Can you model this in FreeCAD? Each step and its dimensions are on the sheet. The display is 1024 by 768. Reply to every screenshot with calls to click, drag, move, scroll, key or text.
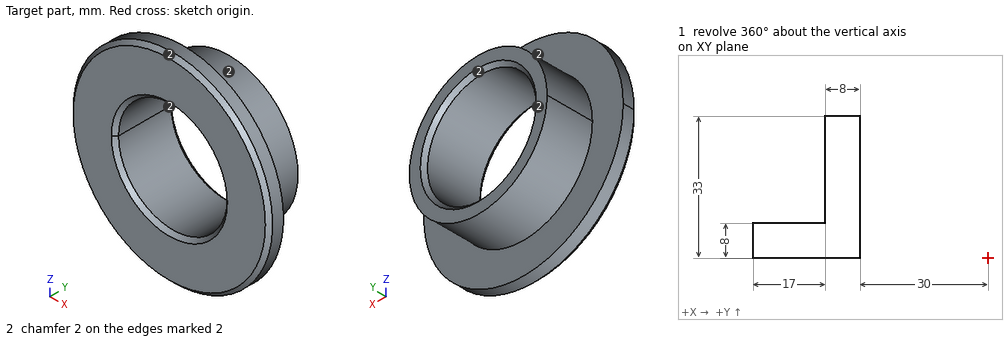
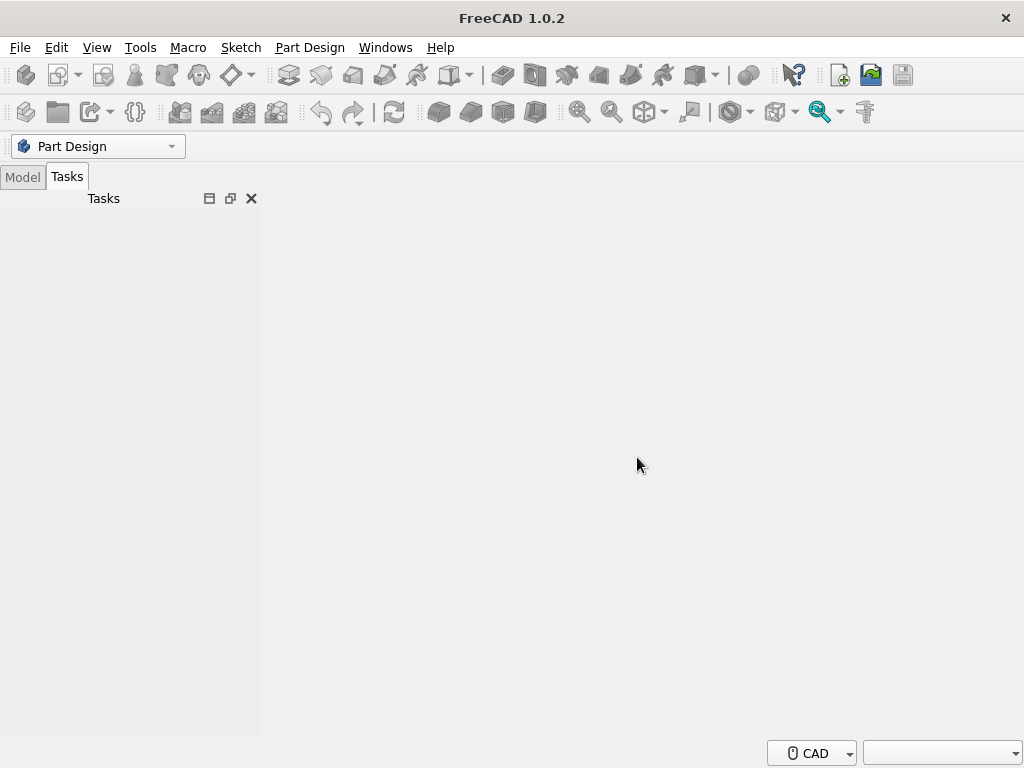
click(840, 76)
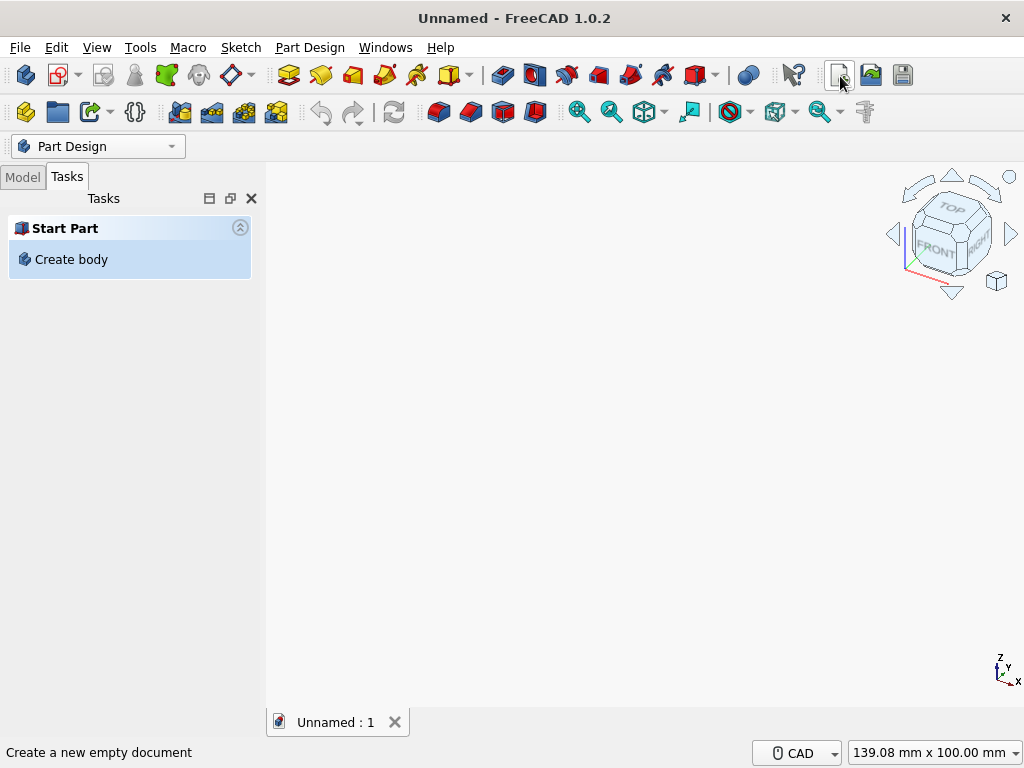
click(58, 76)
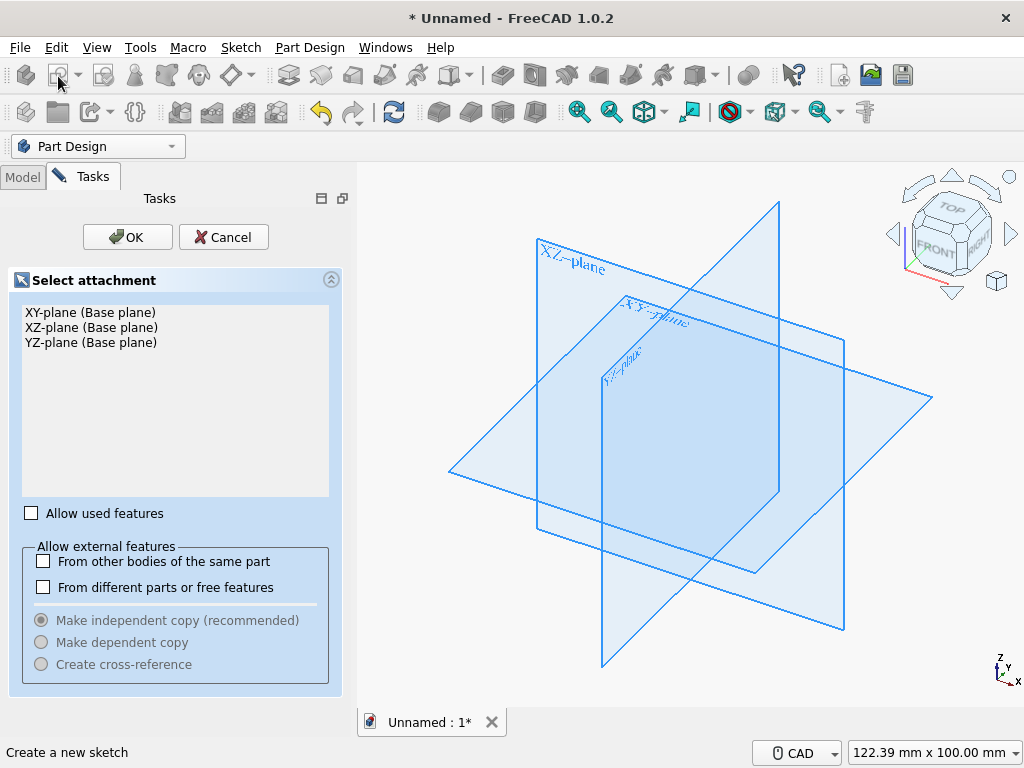
click(82, 312)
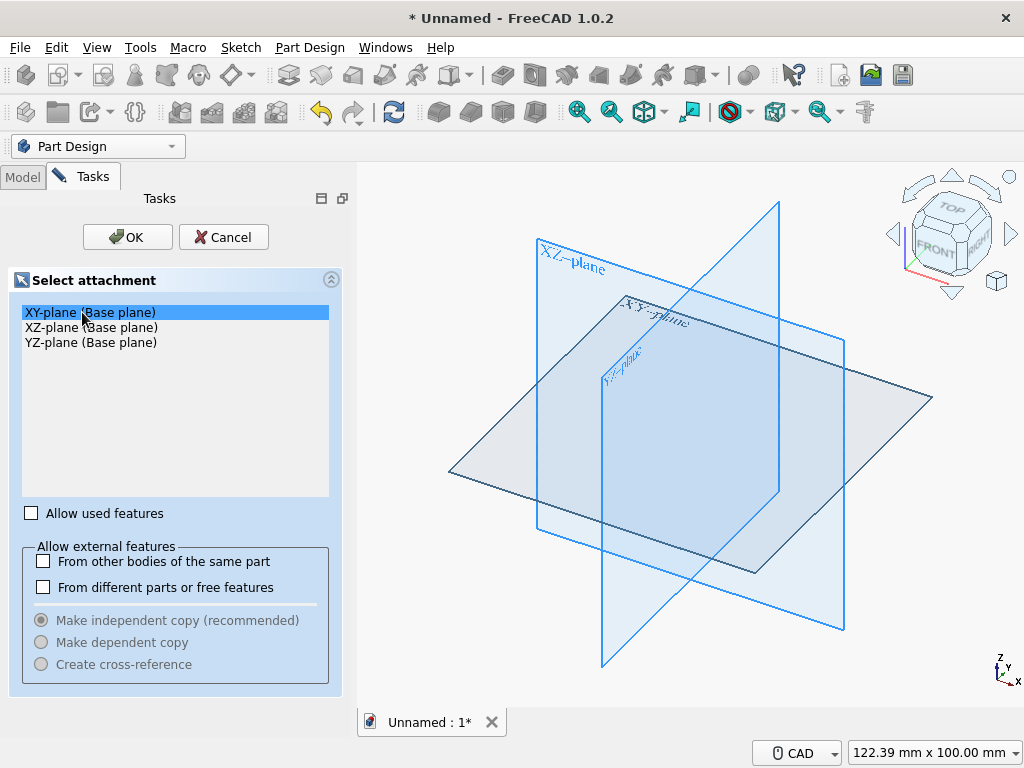
click(128, 237)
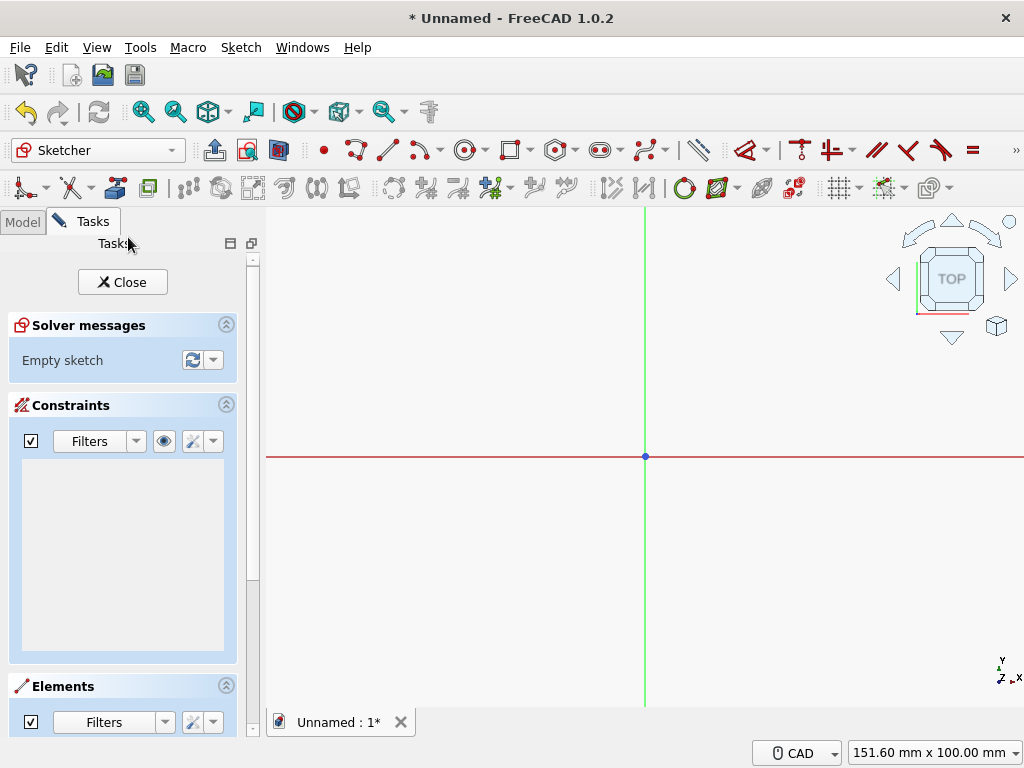
scroll(367, 235, up, 2)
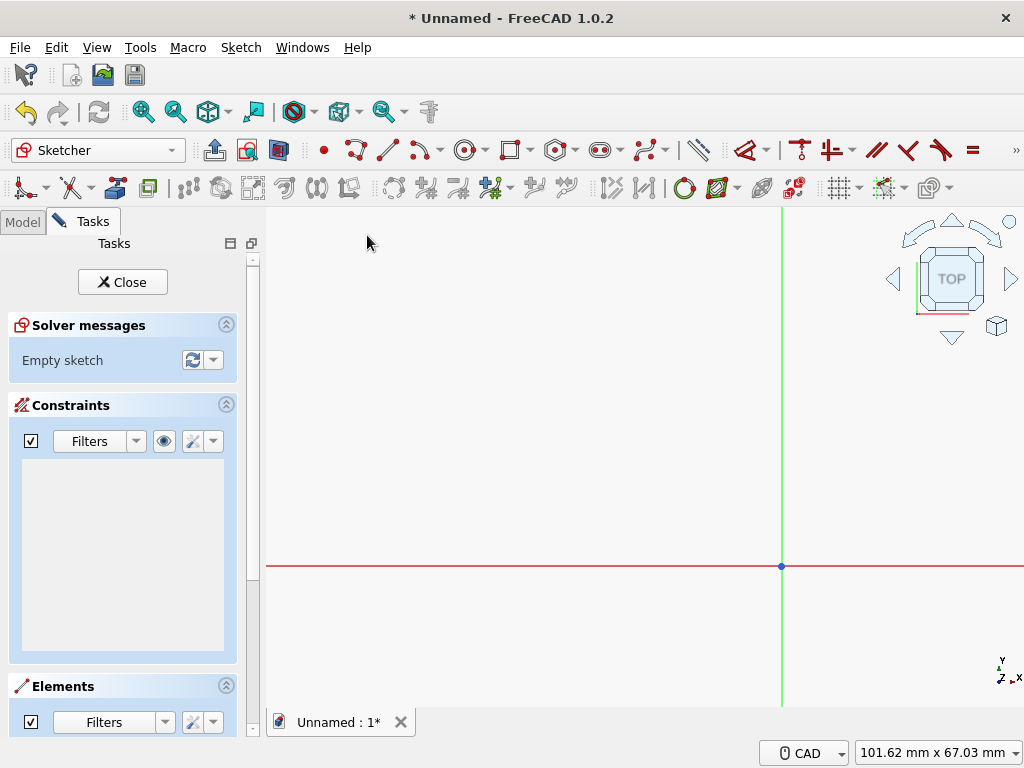
click(356, 150)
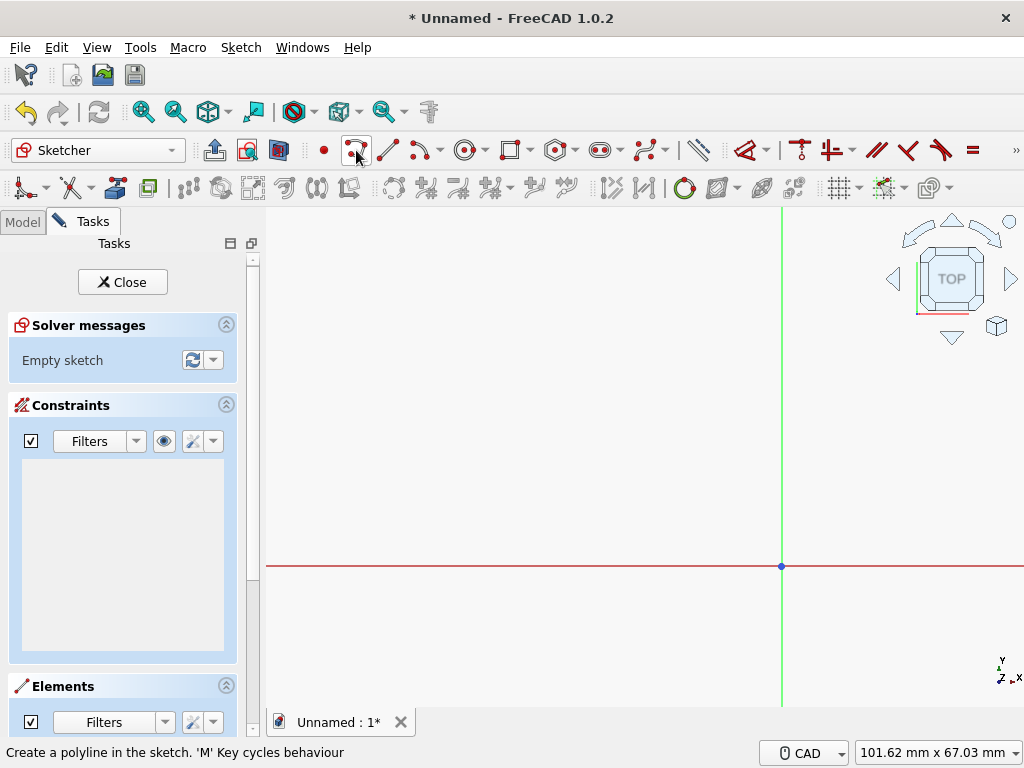
click(558, 566)
click(558, 320)
click(498, 320)
click(498, 506)
click(371, 506)
click(371, 557)
click(558, 566)
key(Escape)
key(Escape)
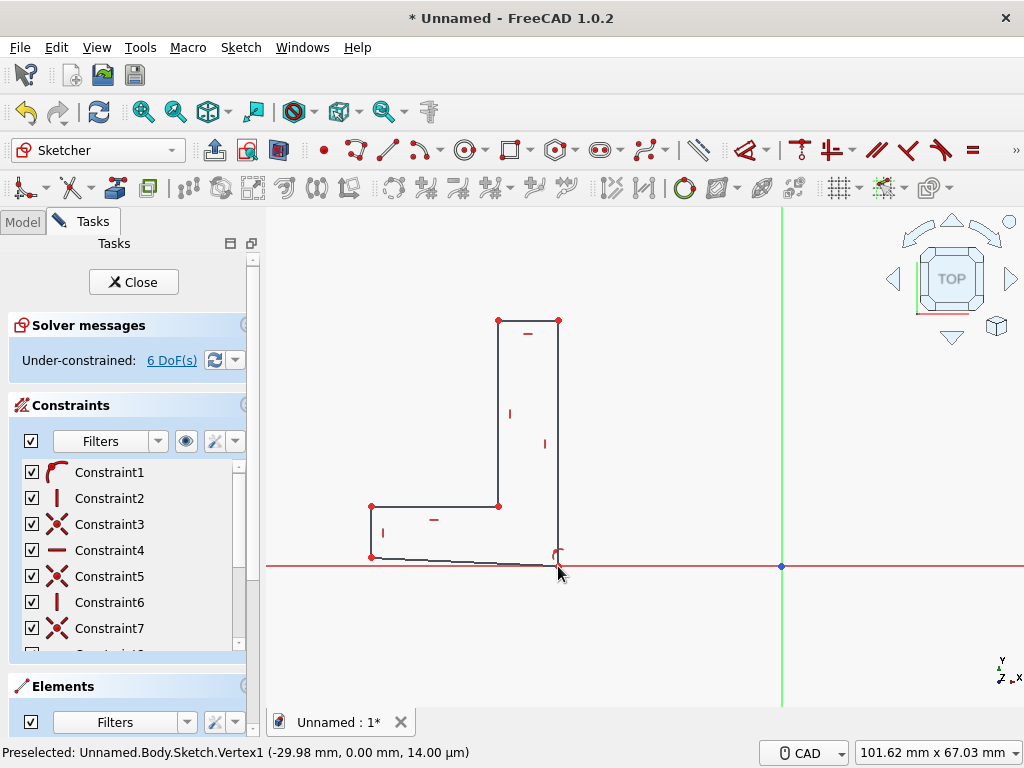
click(502, 564)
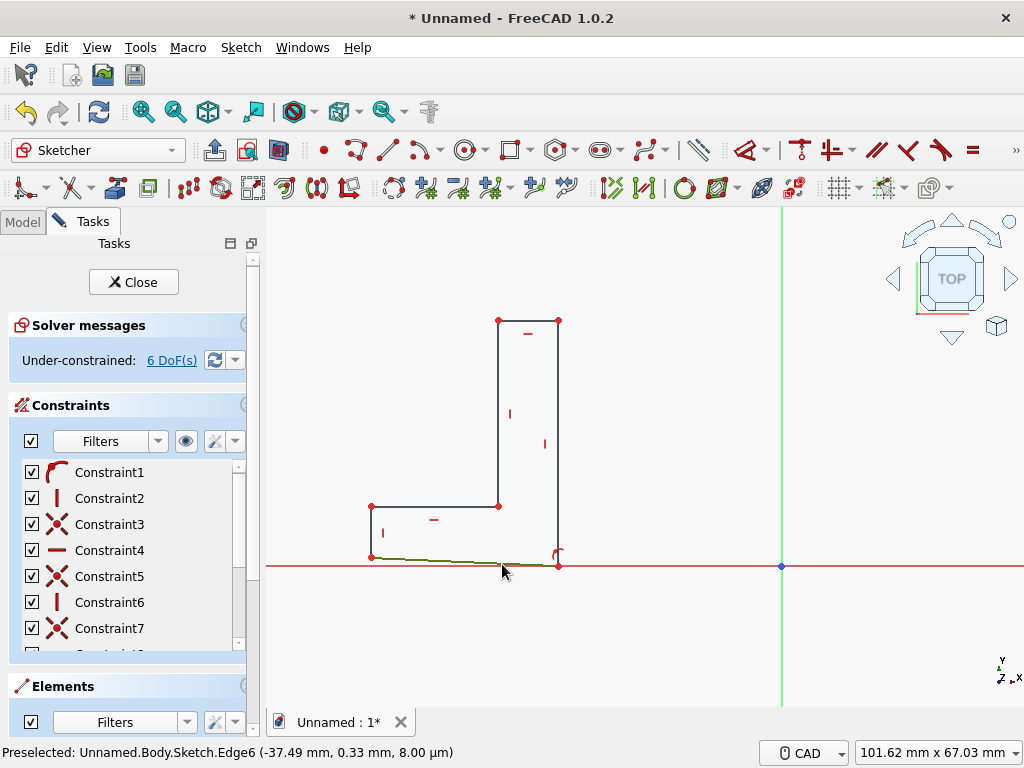
key(h)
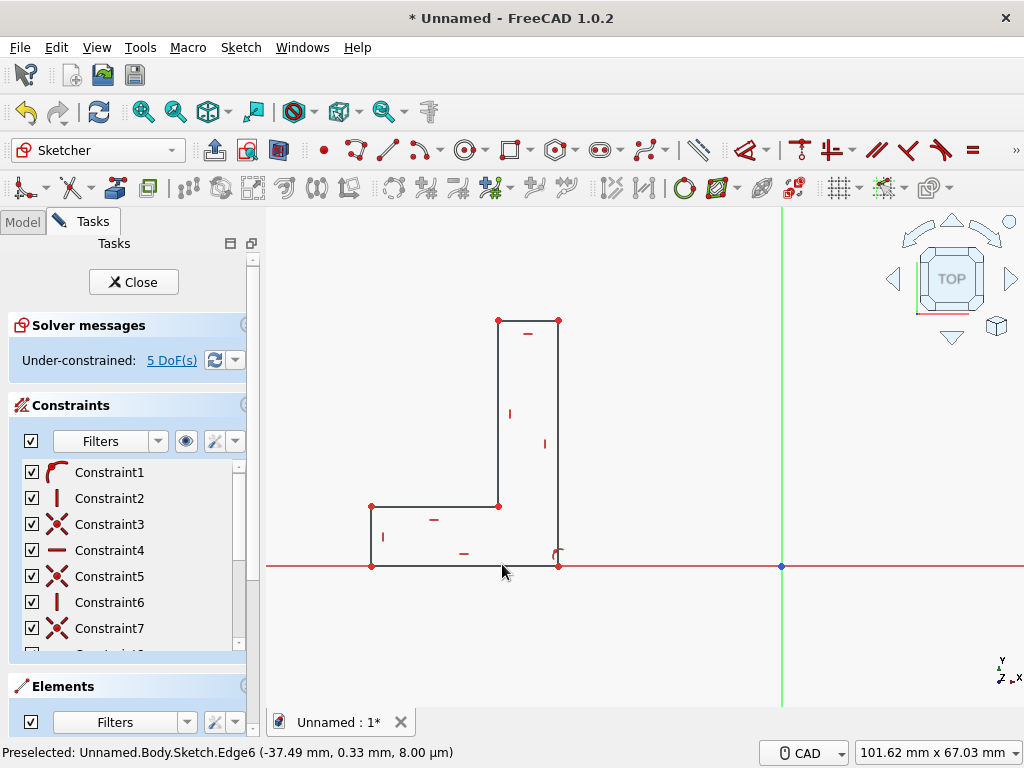
click(746, 150)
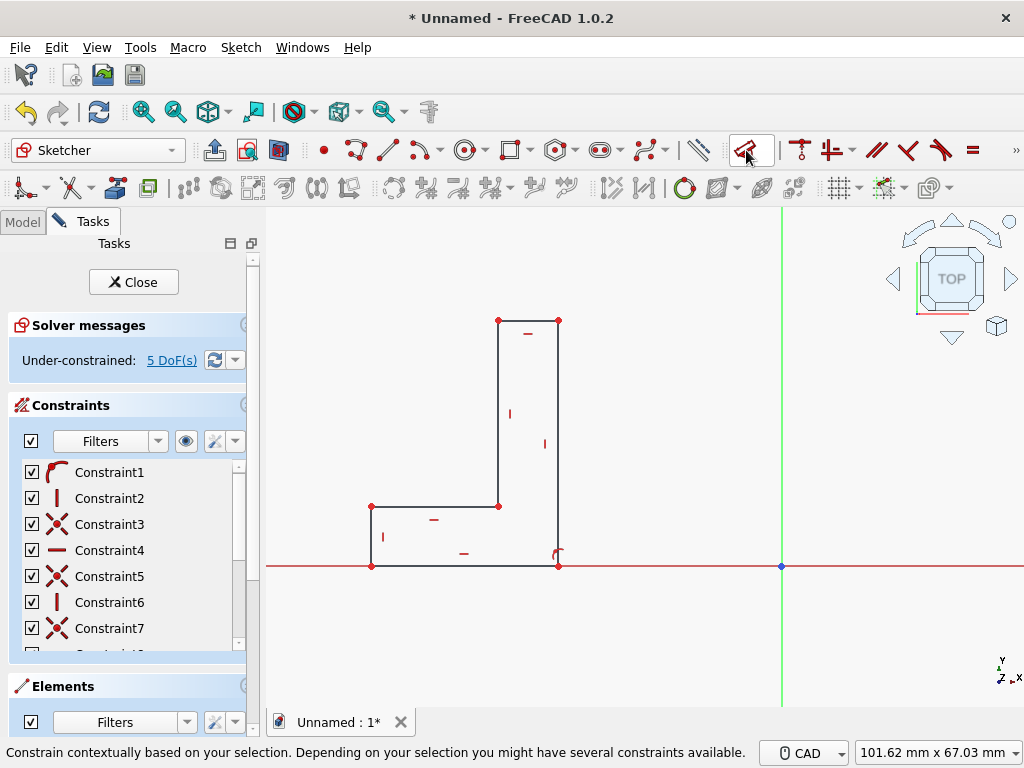
click(540, 321)
click(528, 287)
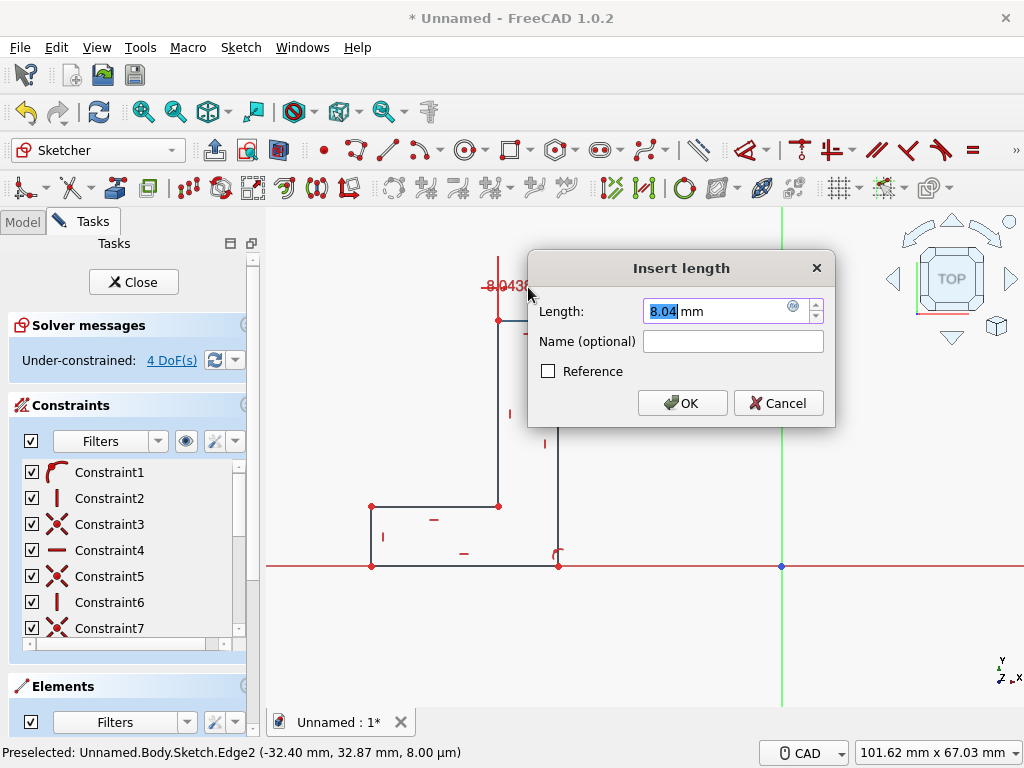
text(8)
key(Return)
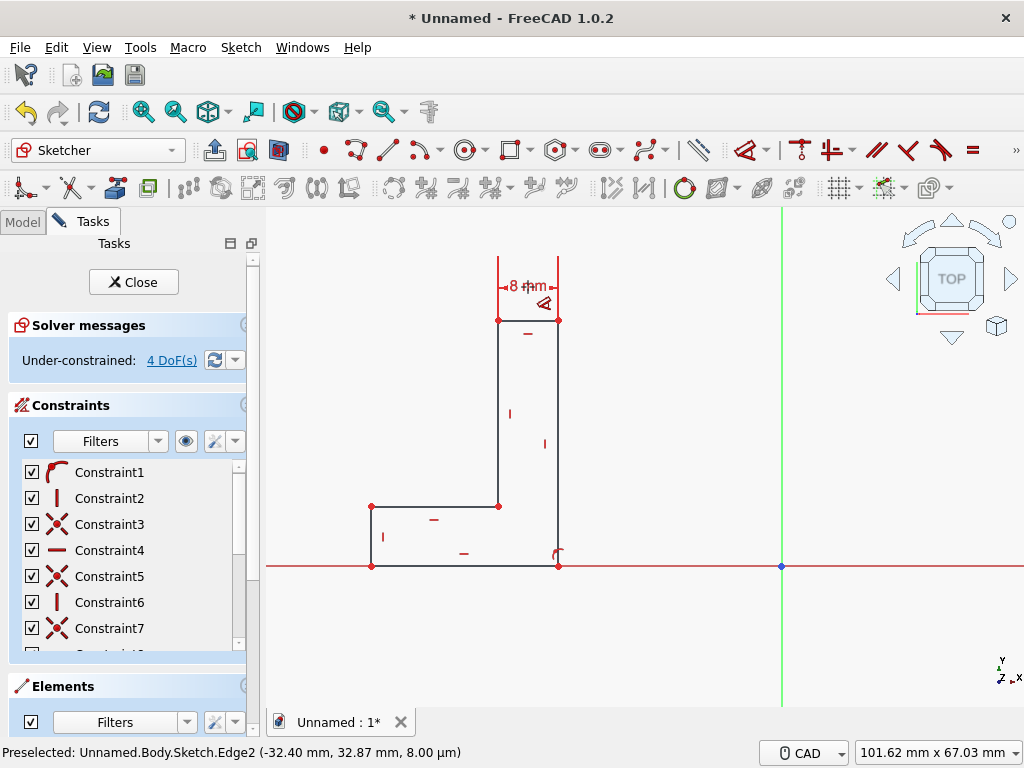
click(371, 525)
click(337, 537)